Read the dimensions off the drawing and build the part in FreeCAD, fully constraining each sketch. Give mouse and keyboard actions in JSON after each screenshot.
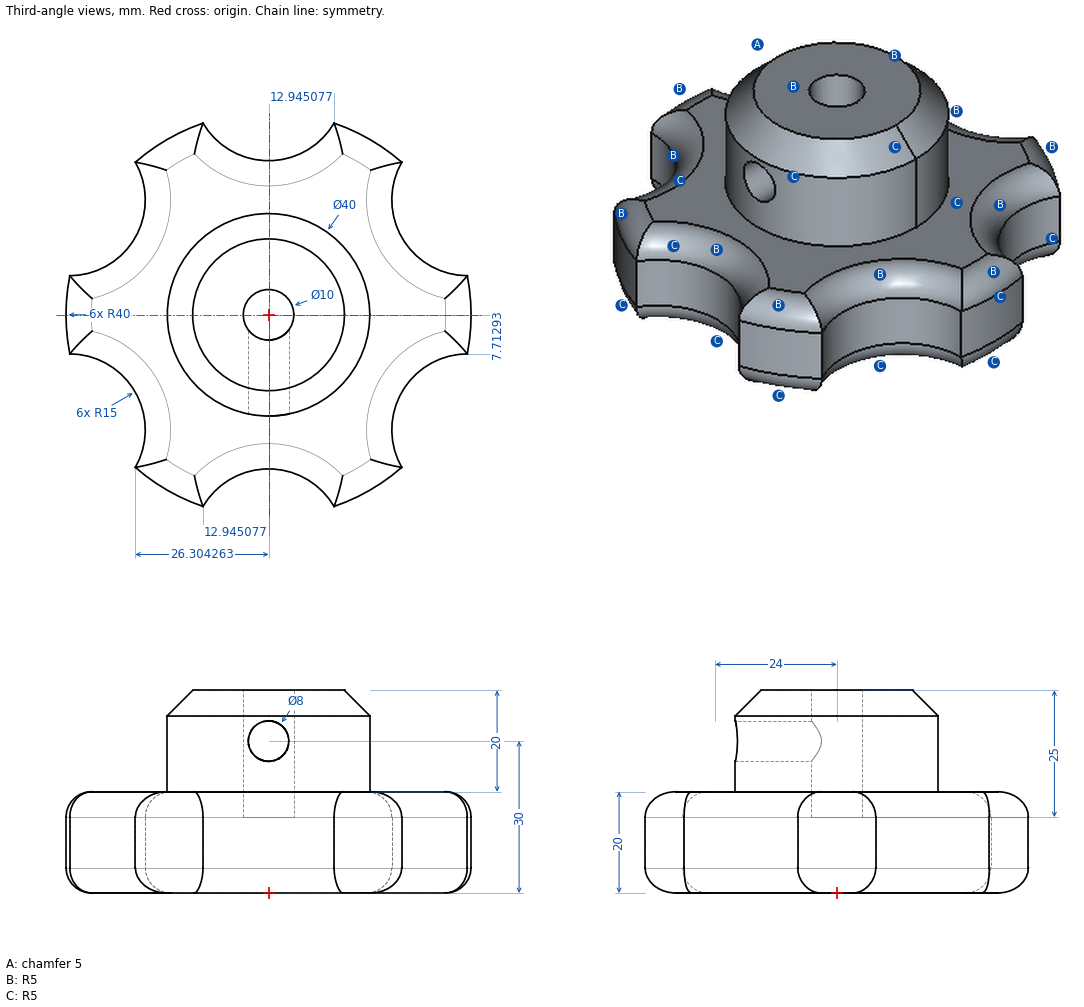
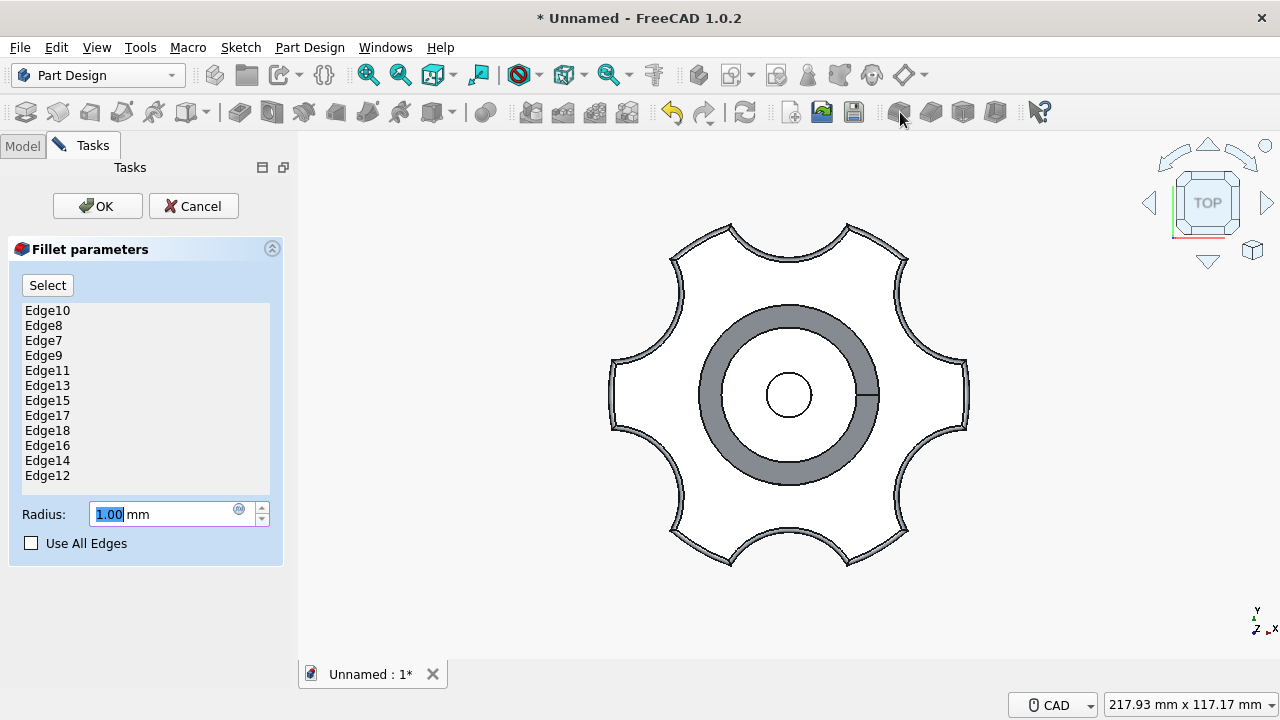
{"action": "type", "text": "5"}
{"action": "key", "text": "Tab"}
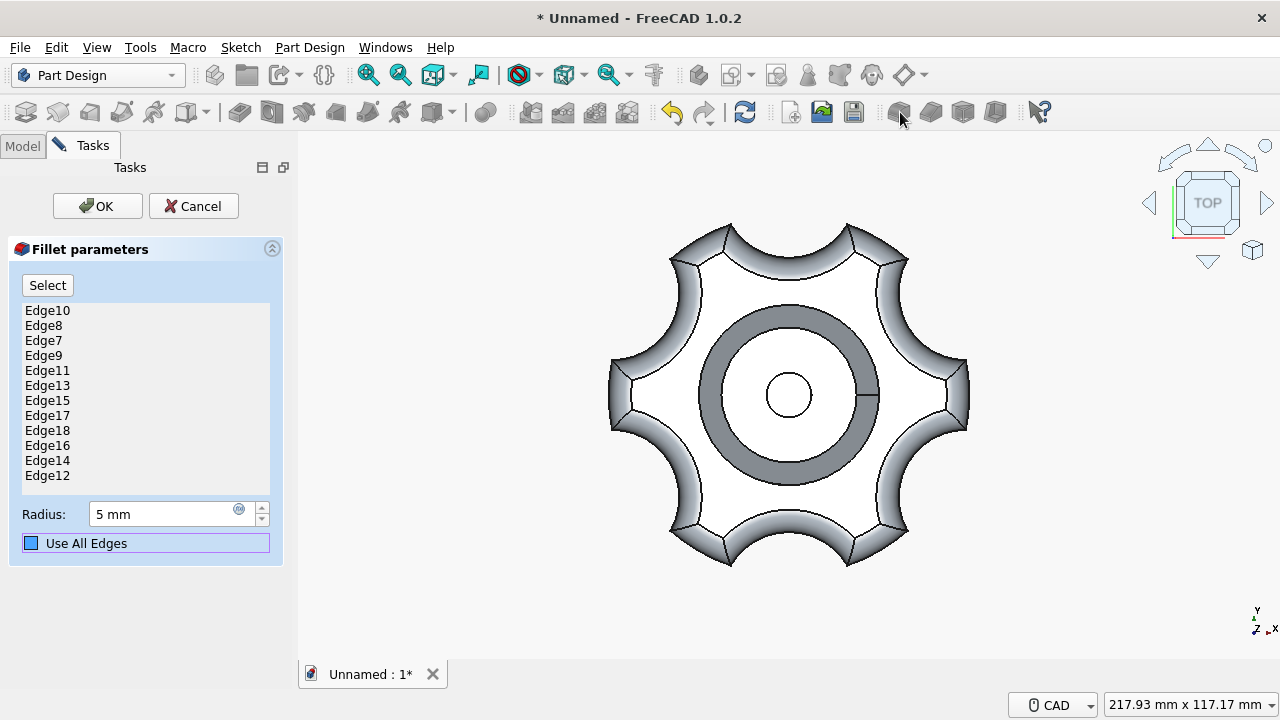
{"action": "left_click", "coordinate": [98, 206]}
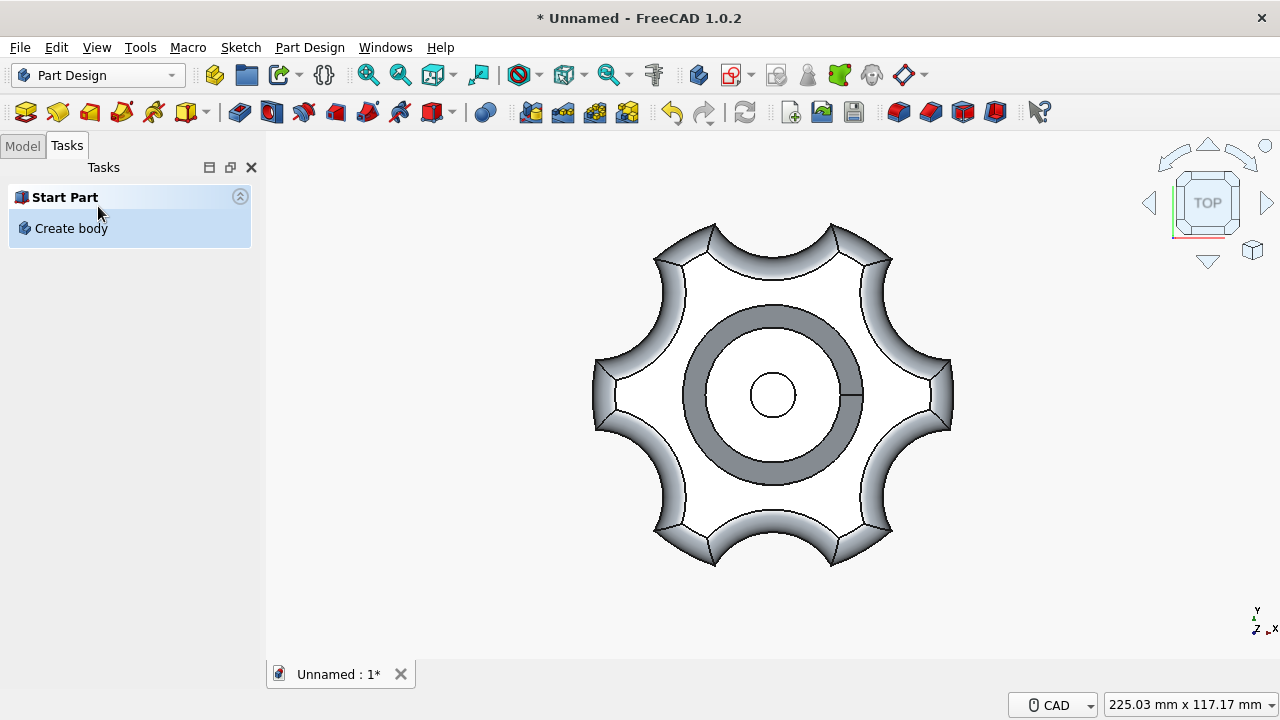
{"action": "key", "text": "0"}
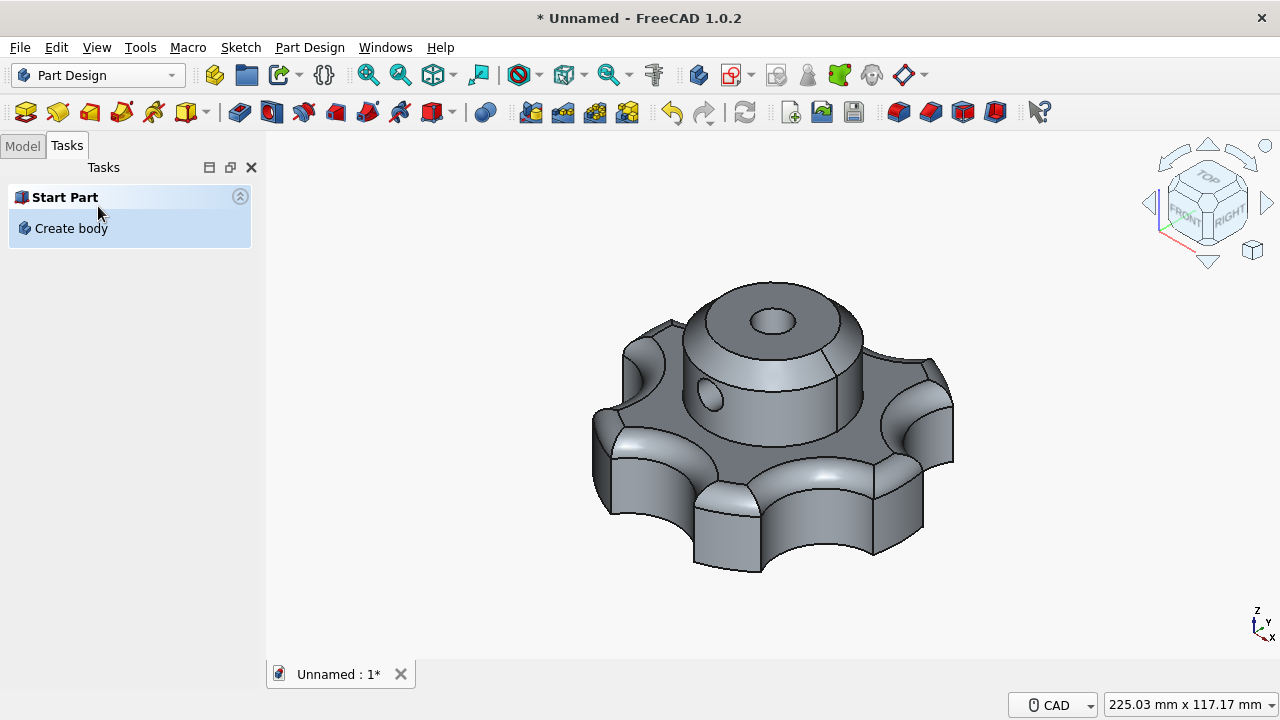
{"action": "key", "text": "2"}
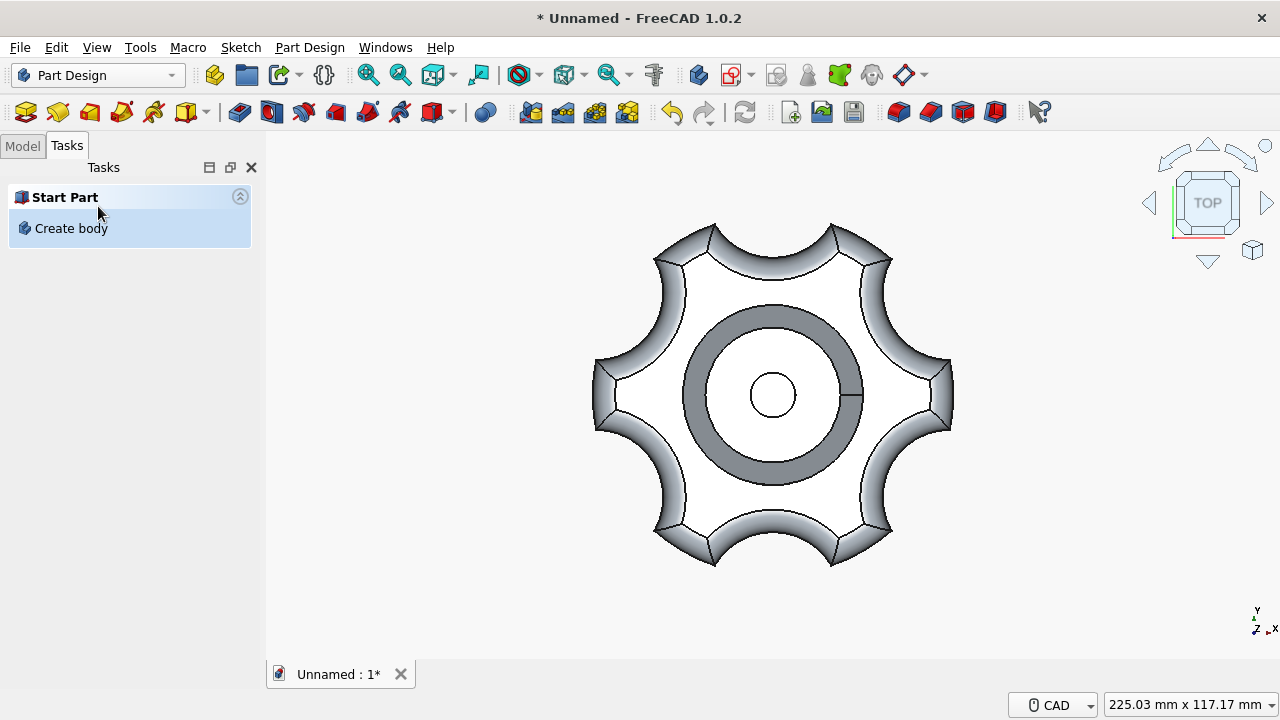
{"action": "key", "text": "1"}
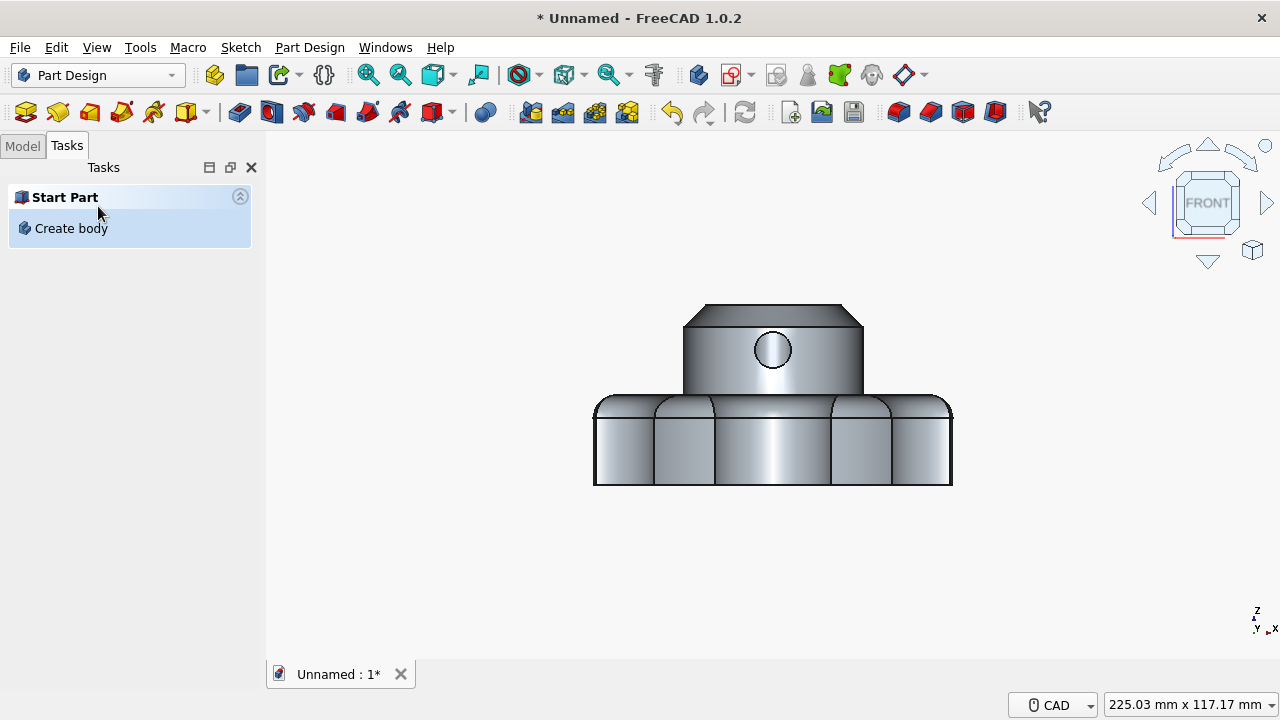
{"action": "left_click", "coordinate": [370, 76]}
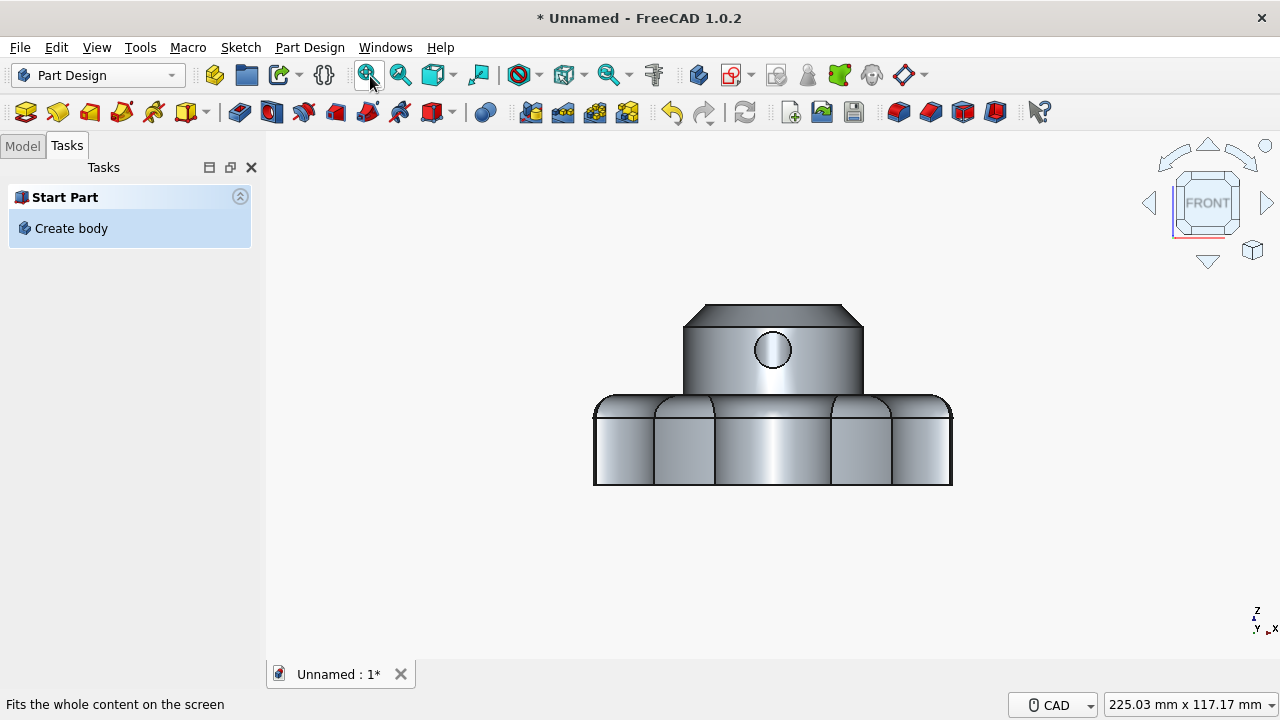
{"action": "key", "text": "3"}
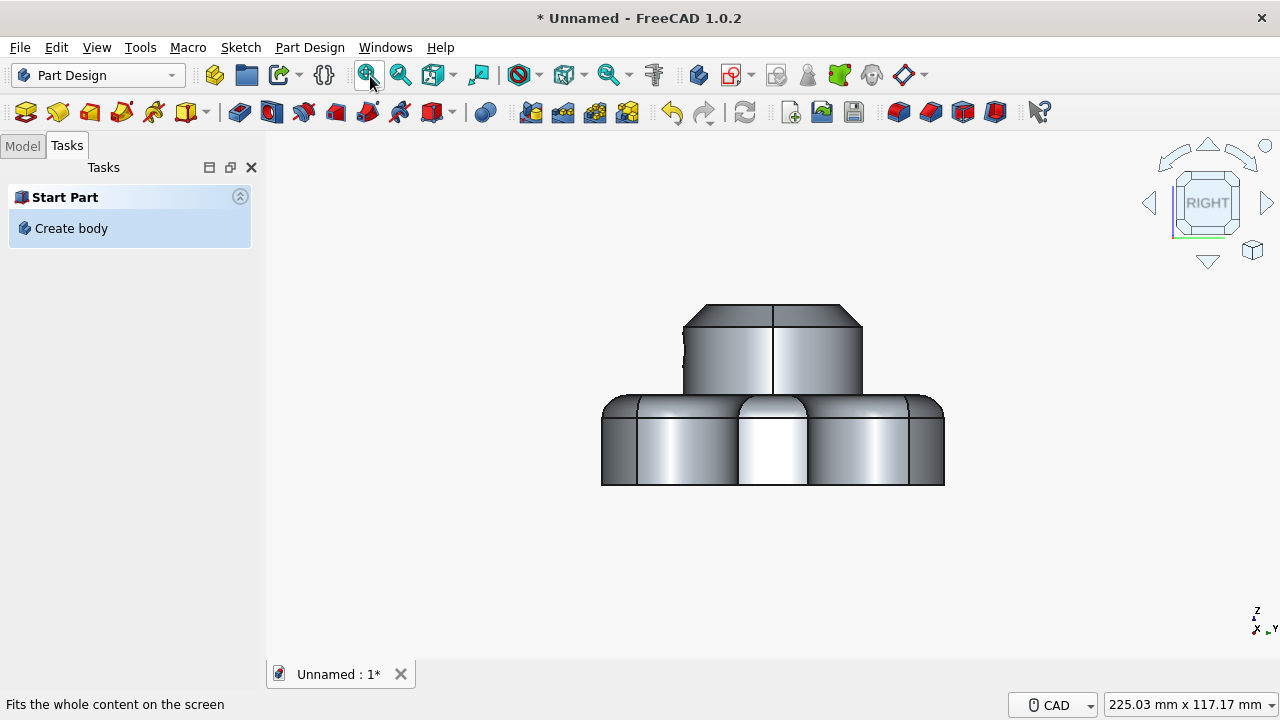
{"action": "left_click", "coordinate": [370, 76]}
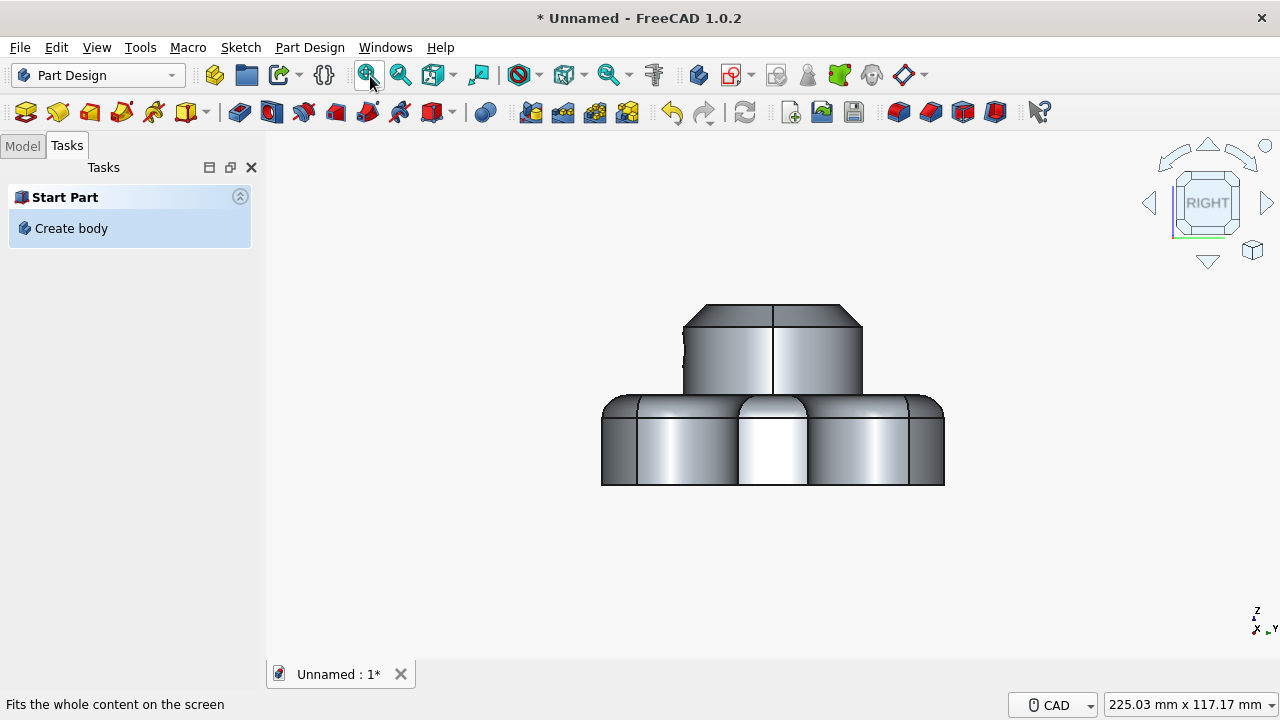
{"action": "key", "text": "5"}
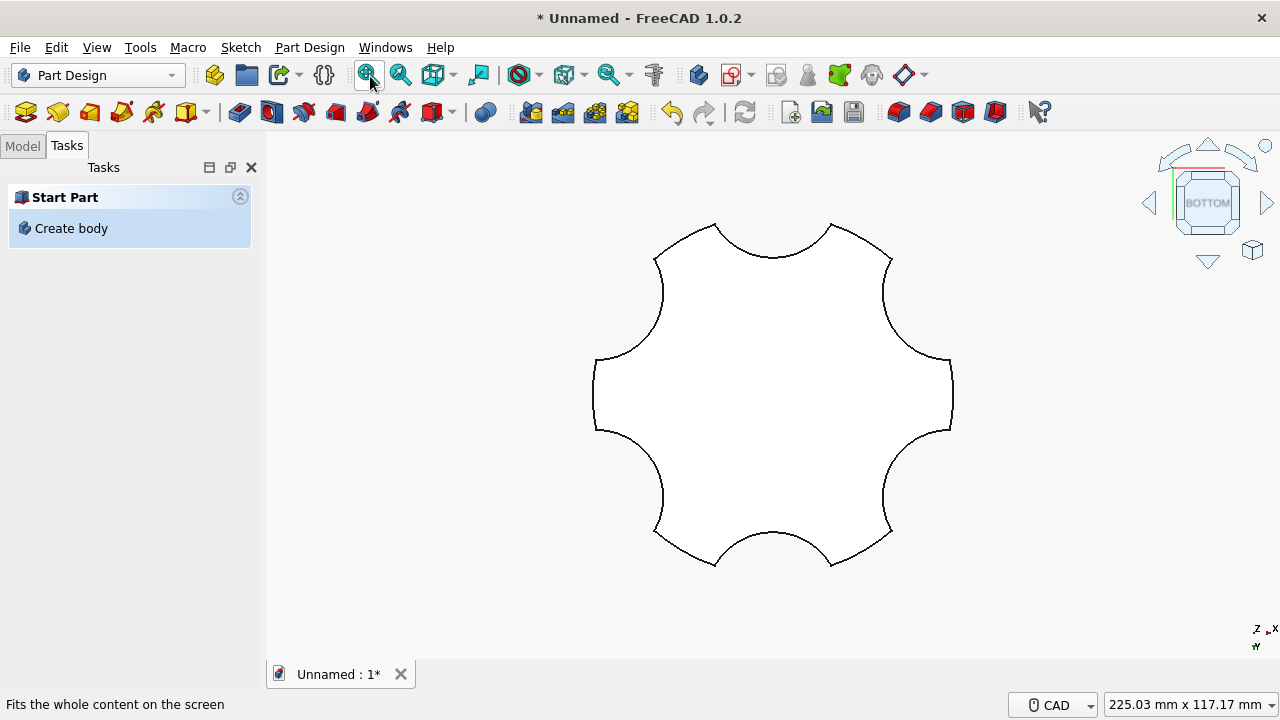
{"action": "left_click", "coordinate": [773, 394]}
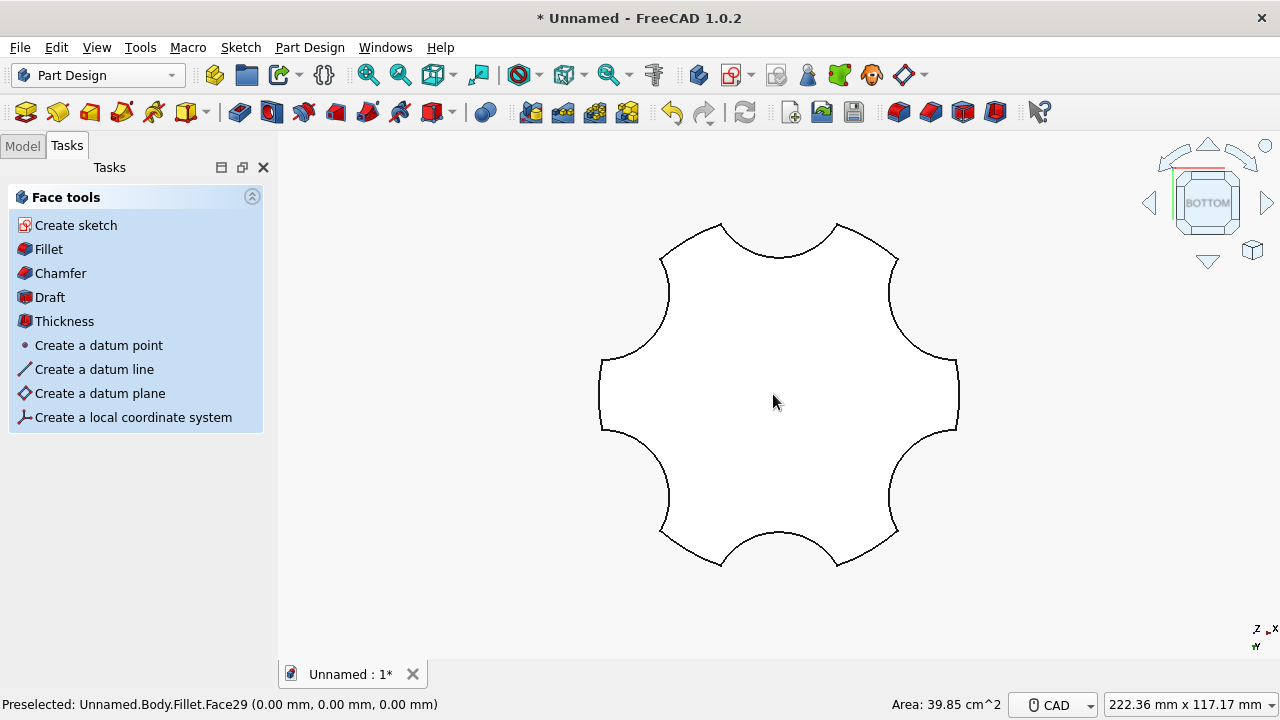
{"action": "left_click", "coordinate": [900, 112]}